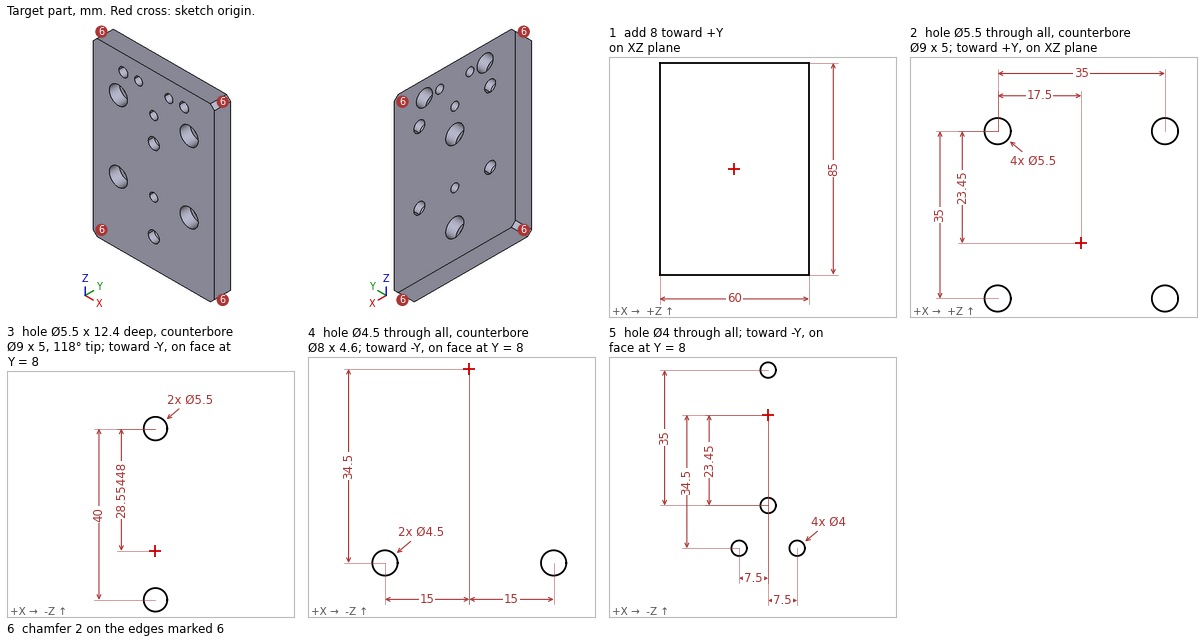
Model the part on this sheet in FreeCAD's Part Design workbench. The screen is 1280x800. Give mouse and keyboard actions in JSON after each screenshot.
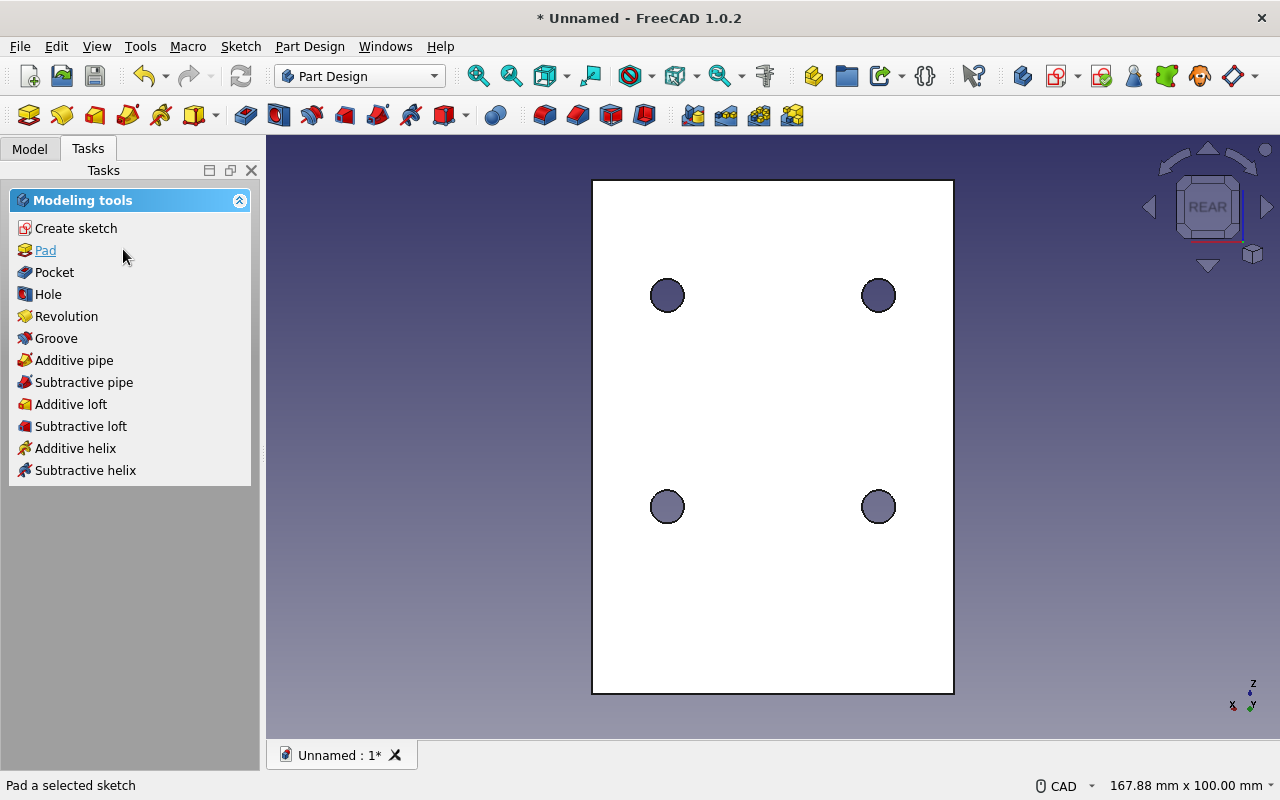
{"action": "left_click", "coordinate": [279, 116]}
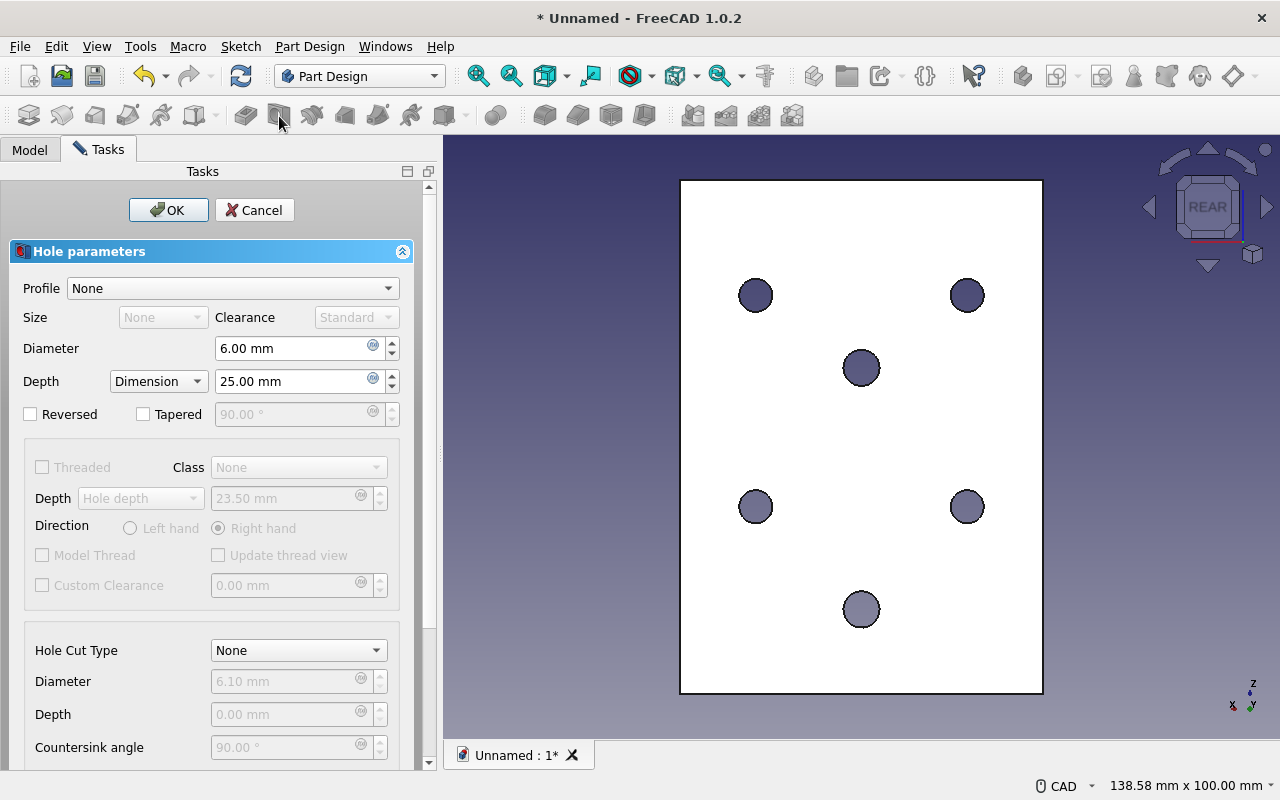
{"action": "triple_click", "coordinate": [300, 348]}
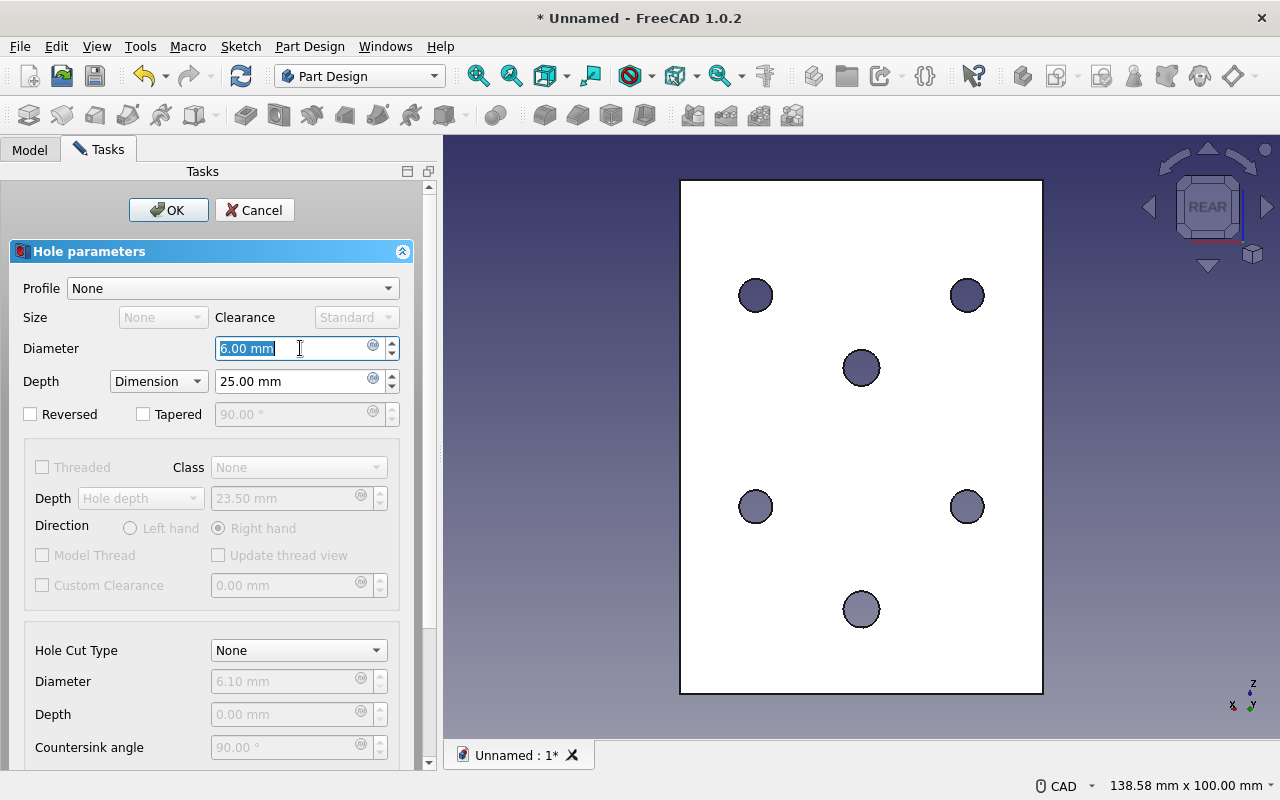
{"action": "type", "text": "5.5"}
{"action": "key", "text": "Tab"}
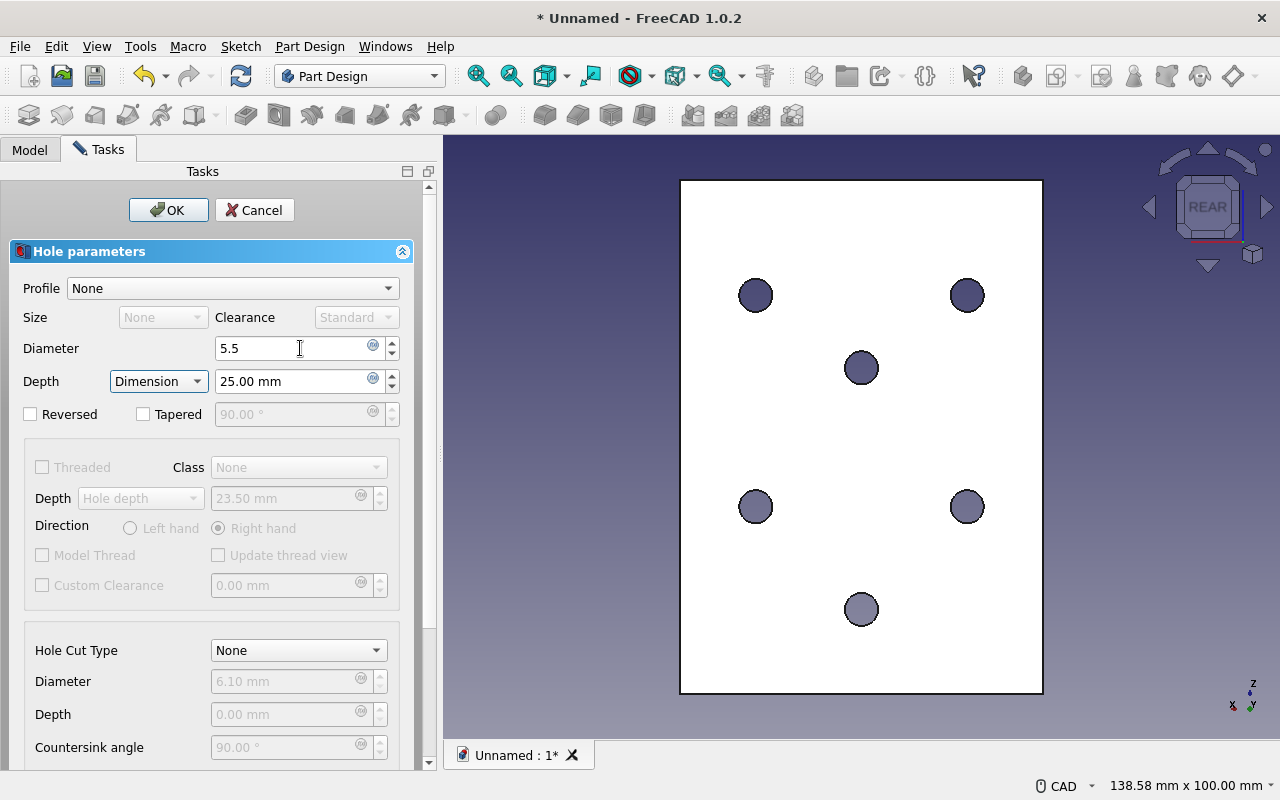
{"action": "triple_click", "coordinate": [300, 382]}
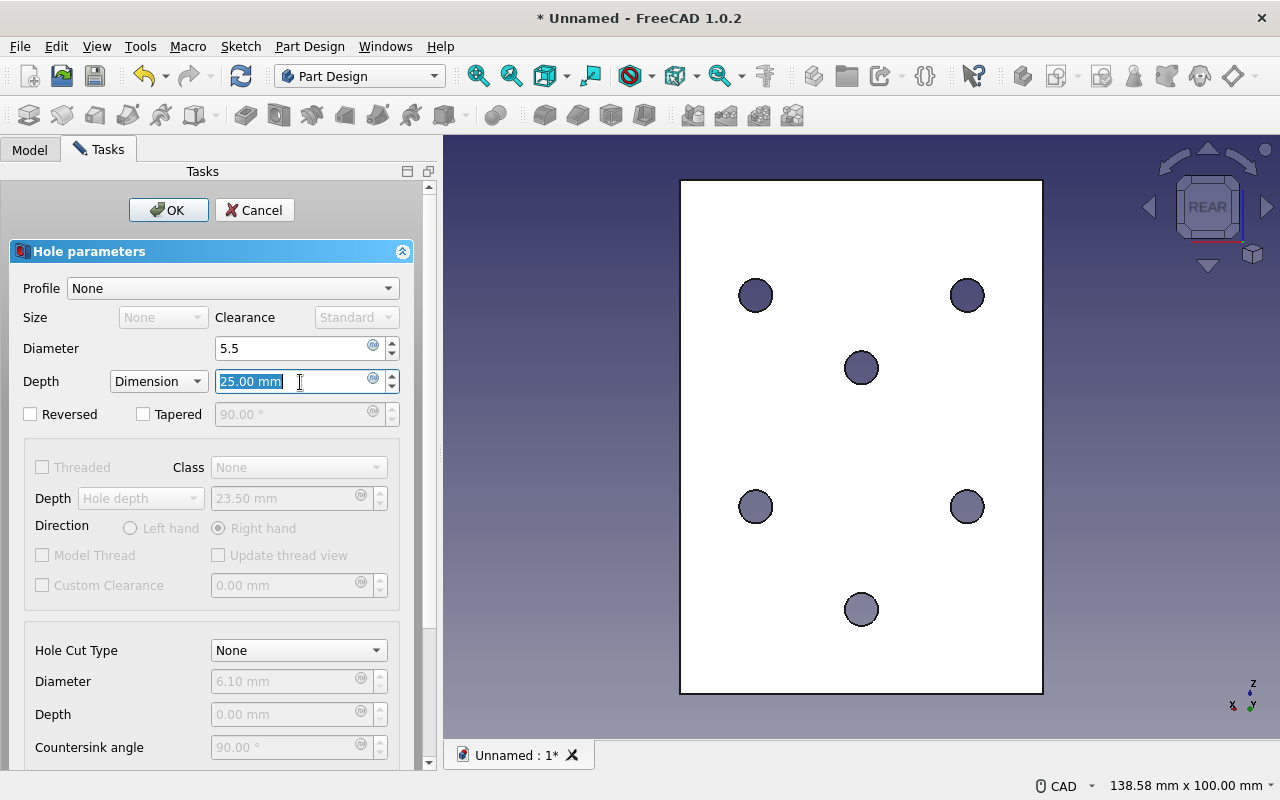
{"action": "type", "text": "12.4"}
{"action": "key", "text": "Tab"}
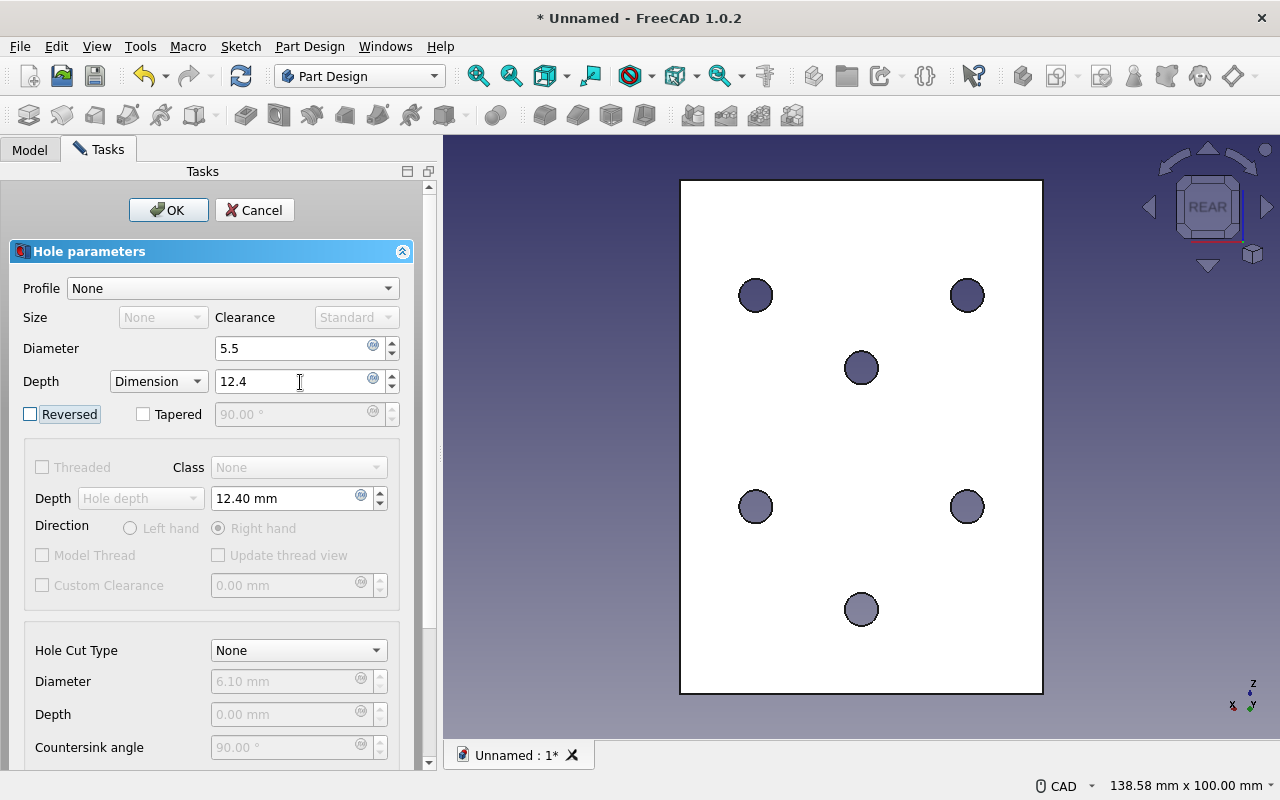
{"action": "left_click", "coordinate": [300, 650]}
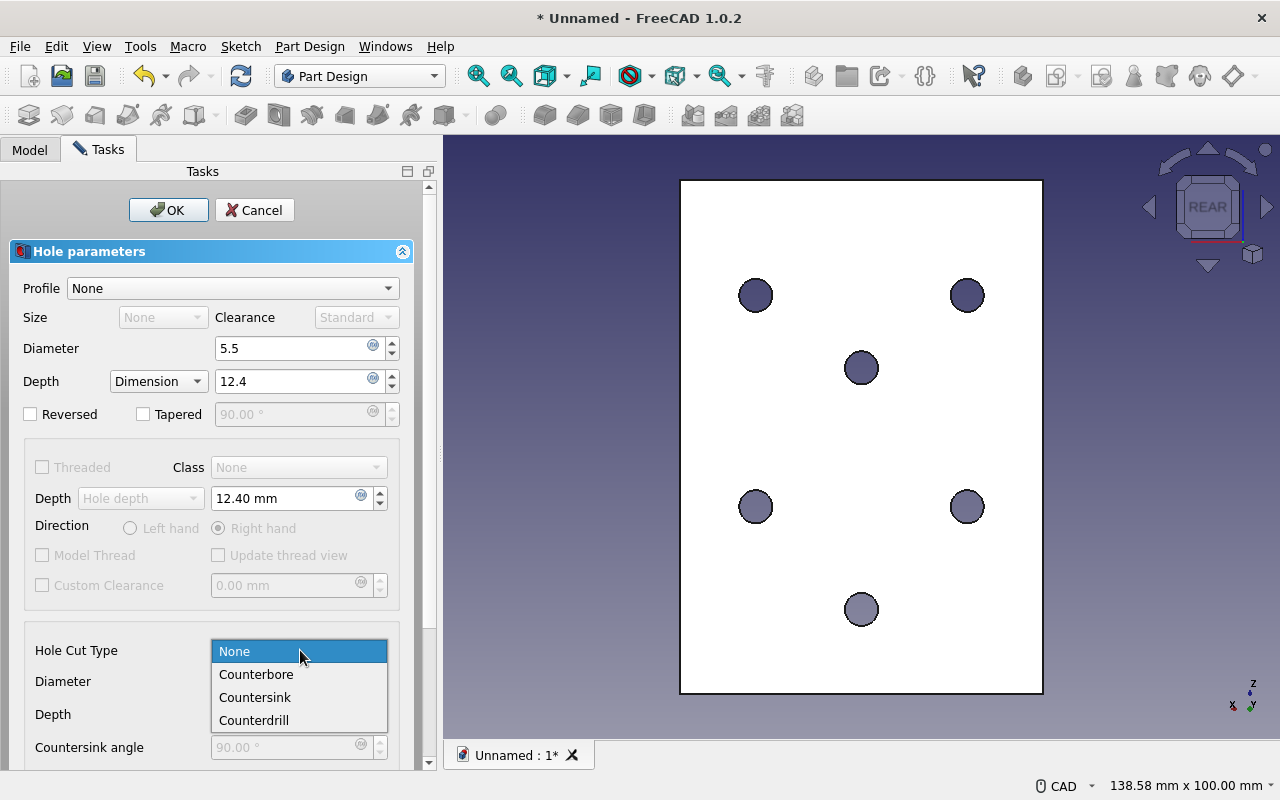
{"action": "left_click", "coordinate": [298, 674]}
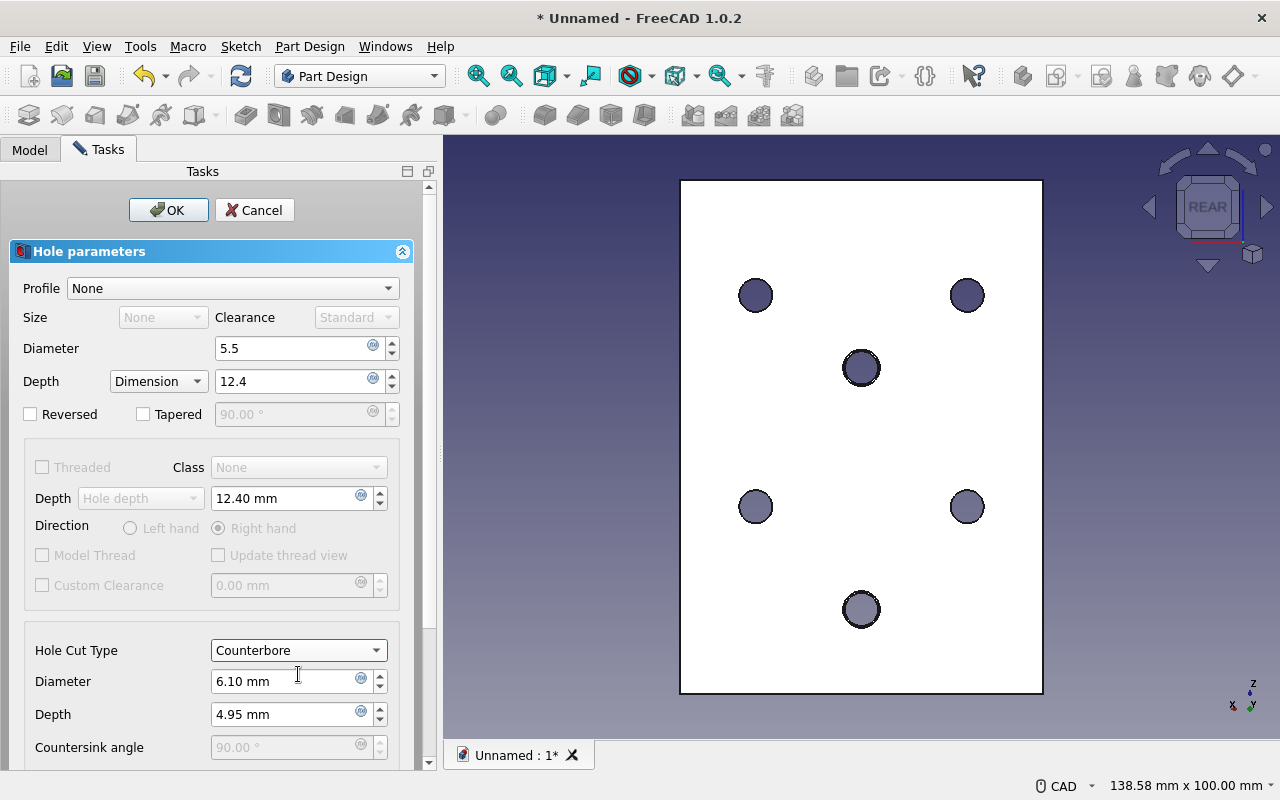
{"action": "triple_click", "coordinate": [292, 682]}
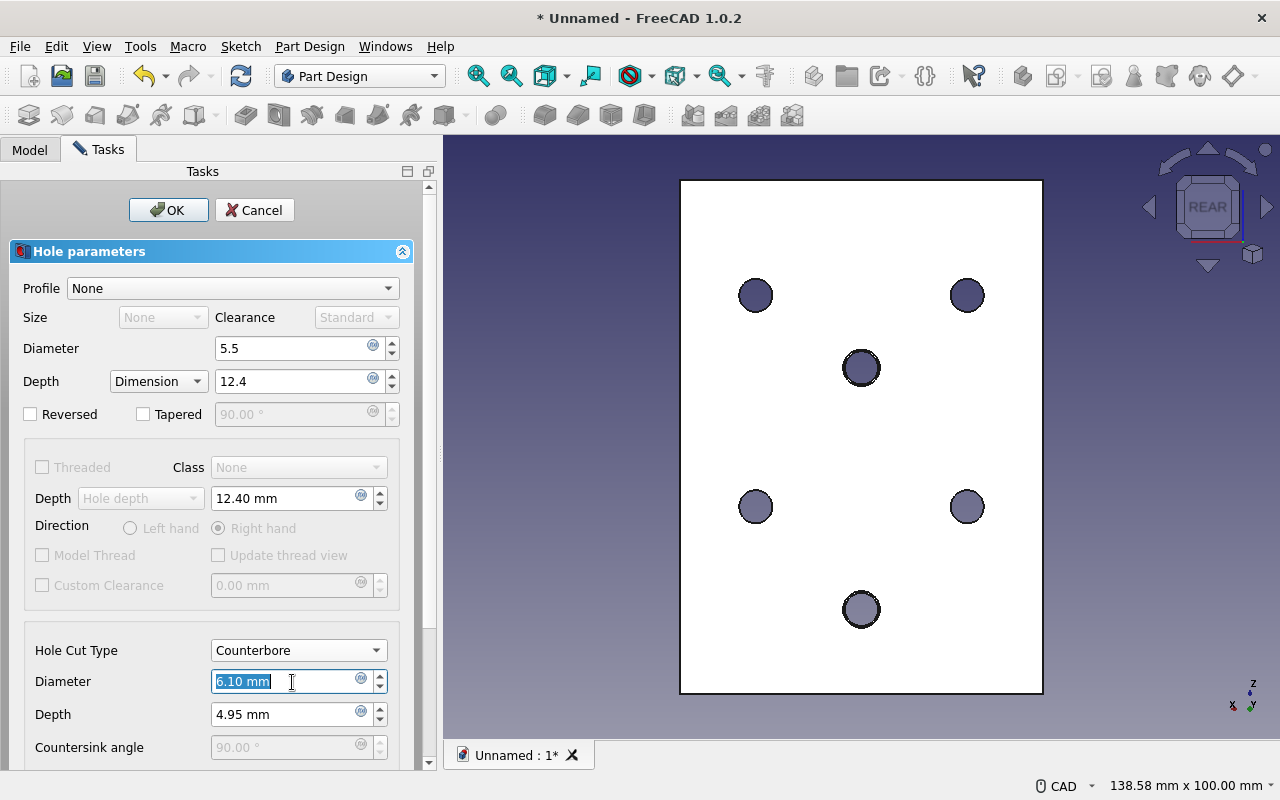
{"action": "type", "text": "9"}
{"action": "key", "text": "Tab"}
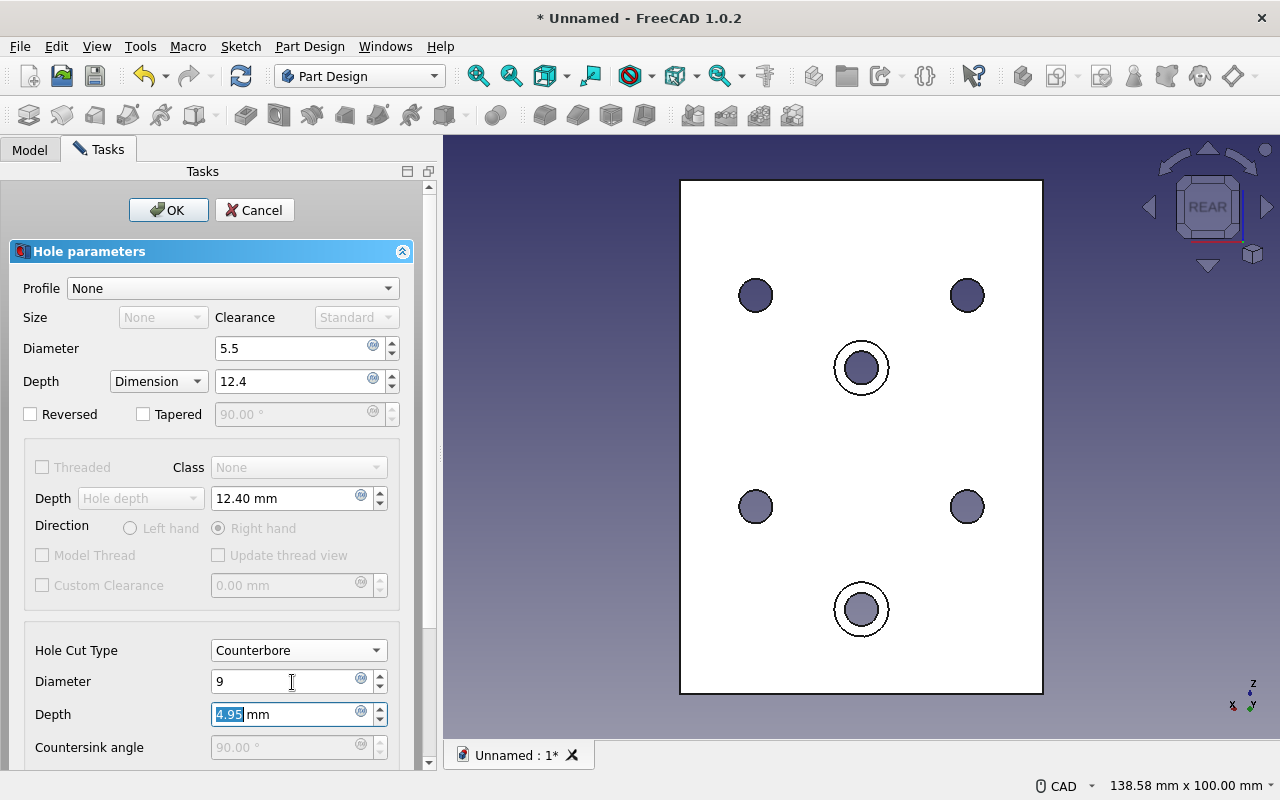
{"action": "type", "text": "5"}
{"action": "key", "text": "Tab"}